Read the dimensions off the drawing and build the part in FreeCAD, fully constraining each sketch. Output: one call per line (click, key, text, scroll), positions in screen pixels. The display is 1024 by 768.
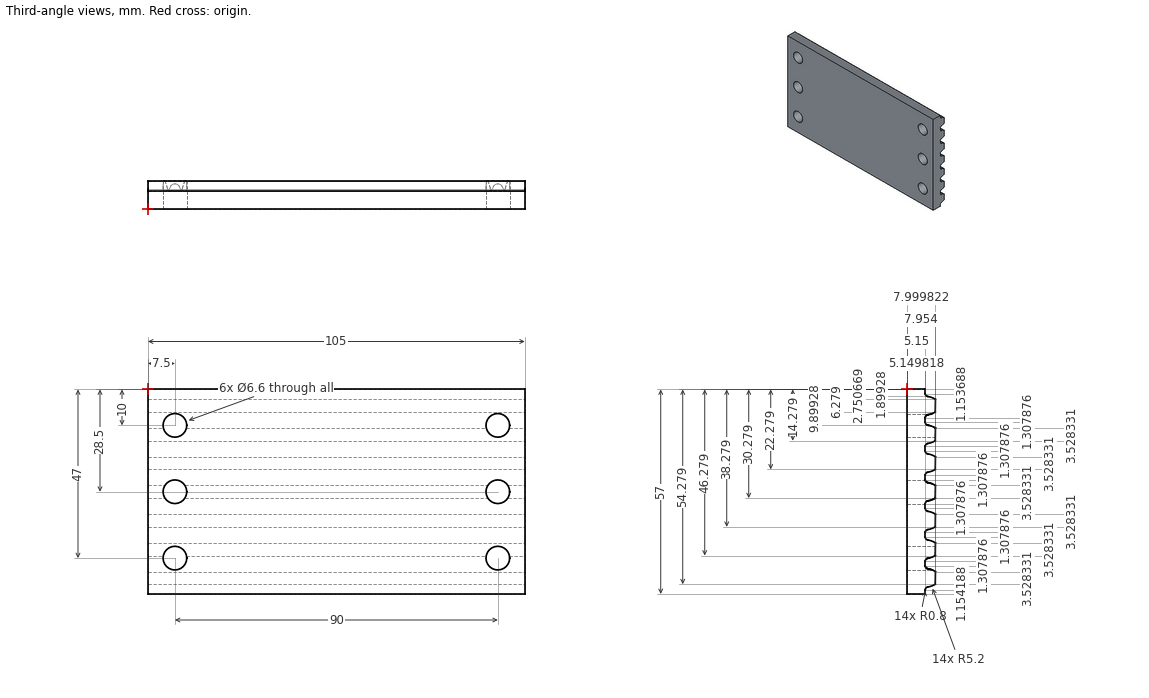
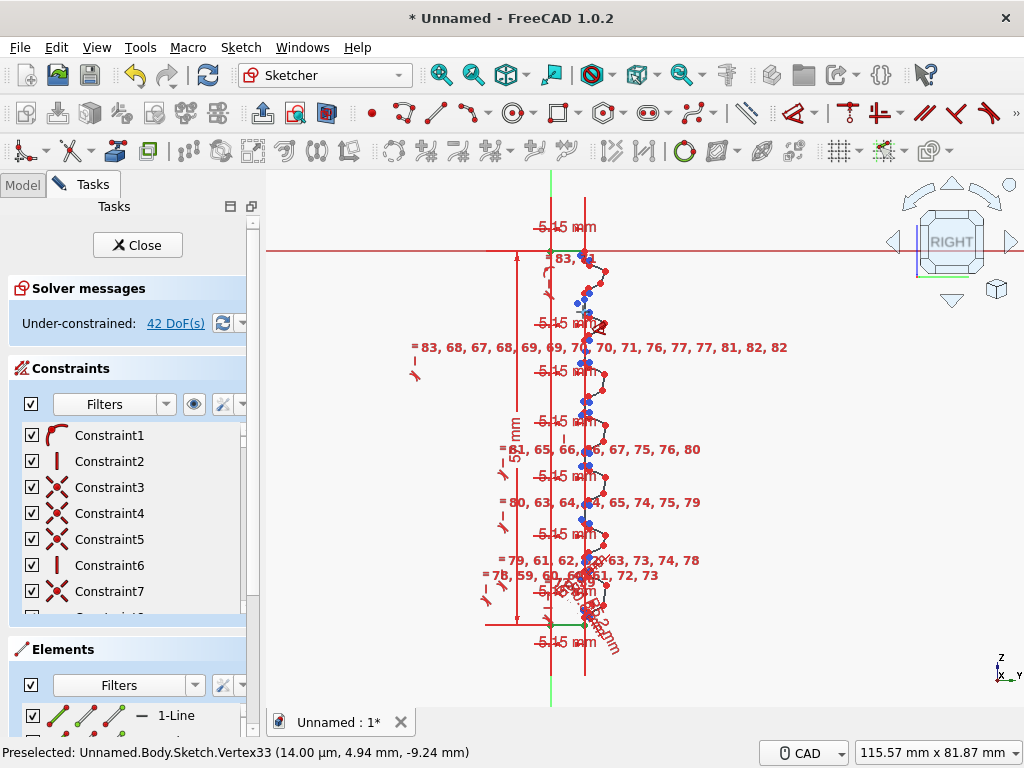
click(603, 605)
click(577, 217)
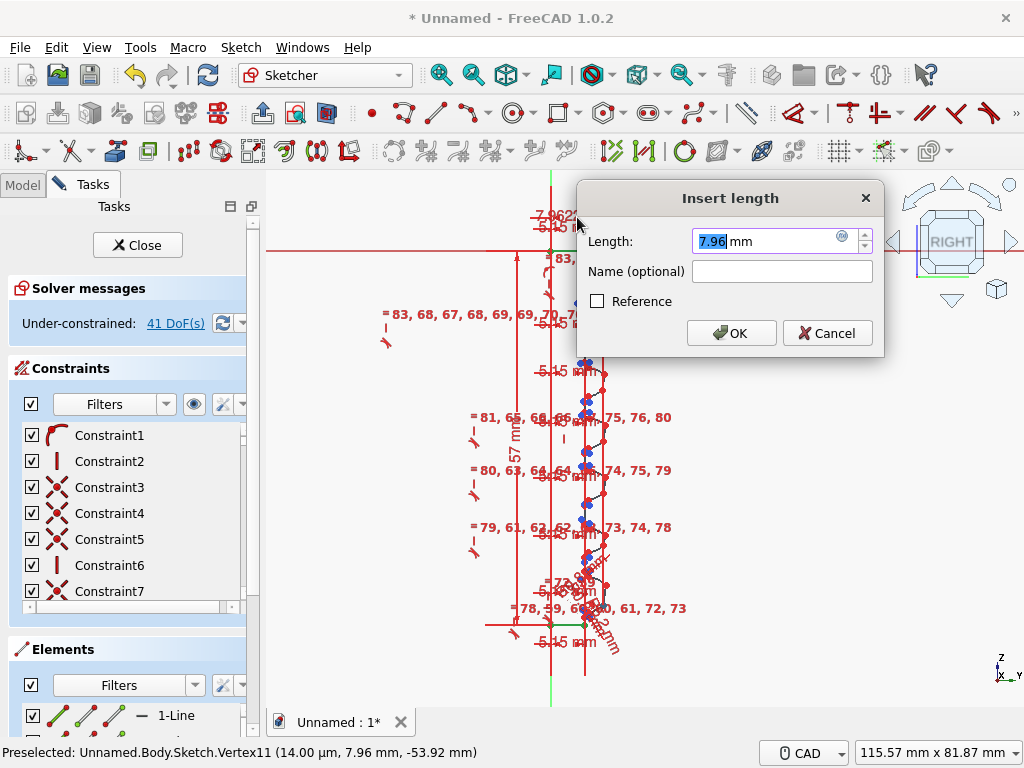
text(7.954)
key(Return)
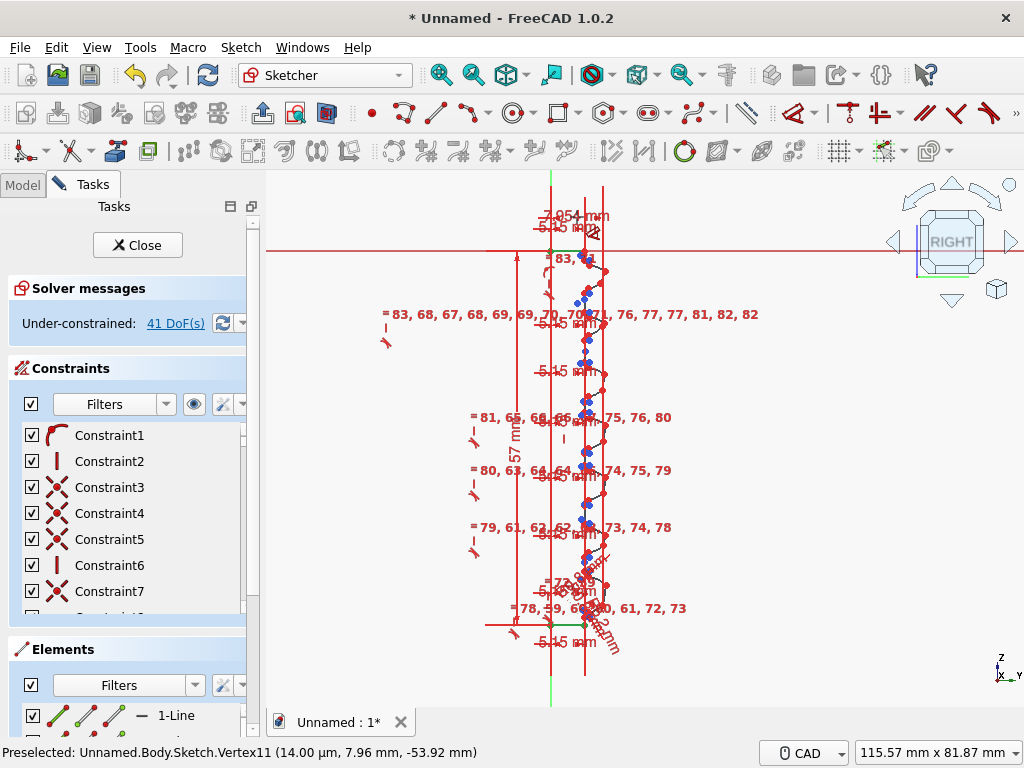
click(603, 546)
click(577, 676)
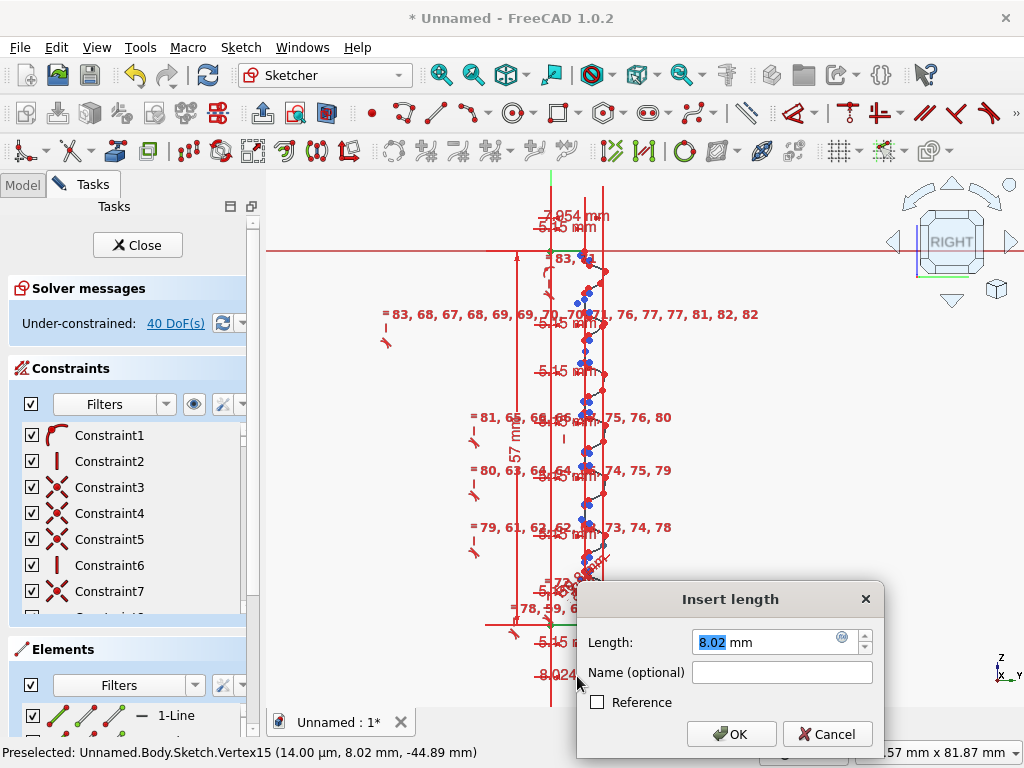
text(7.954)
key(Return)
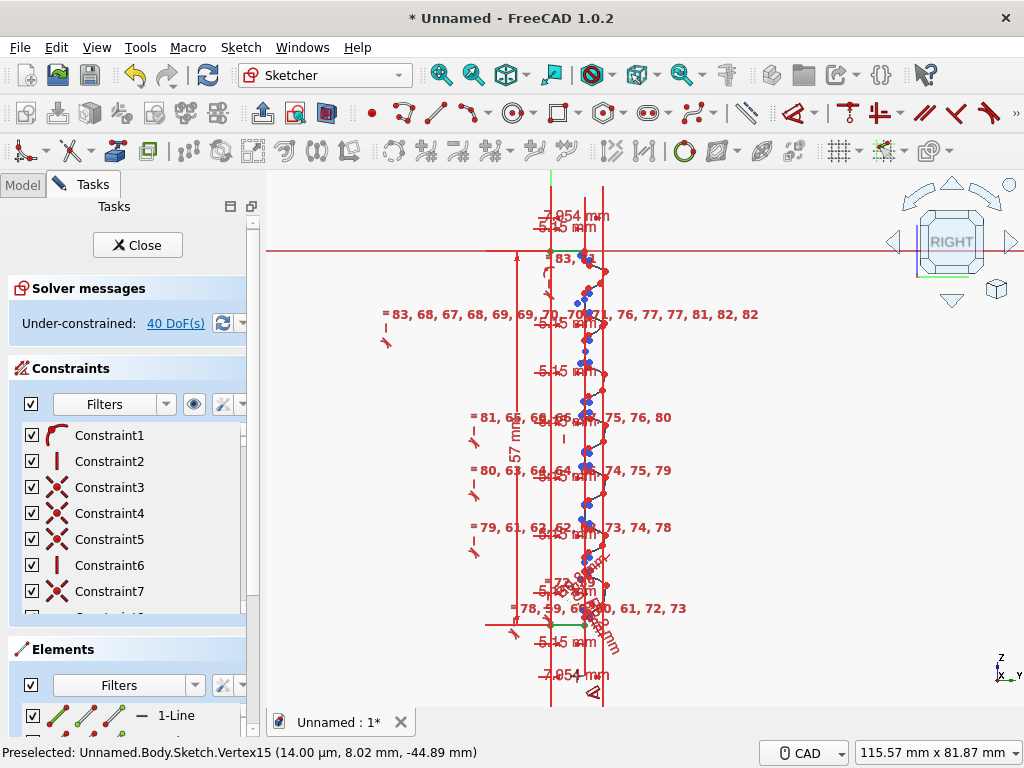
click(603, 493)
click(577, 551)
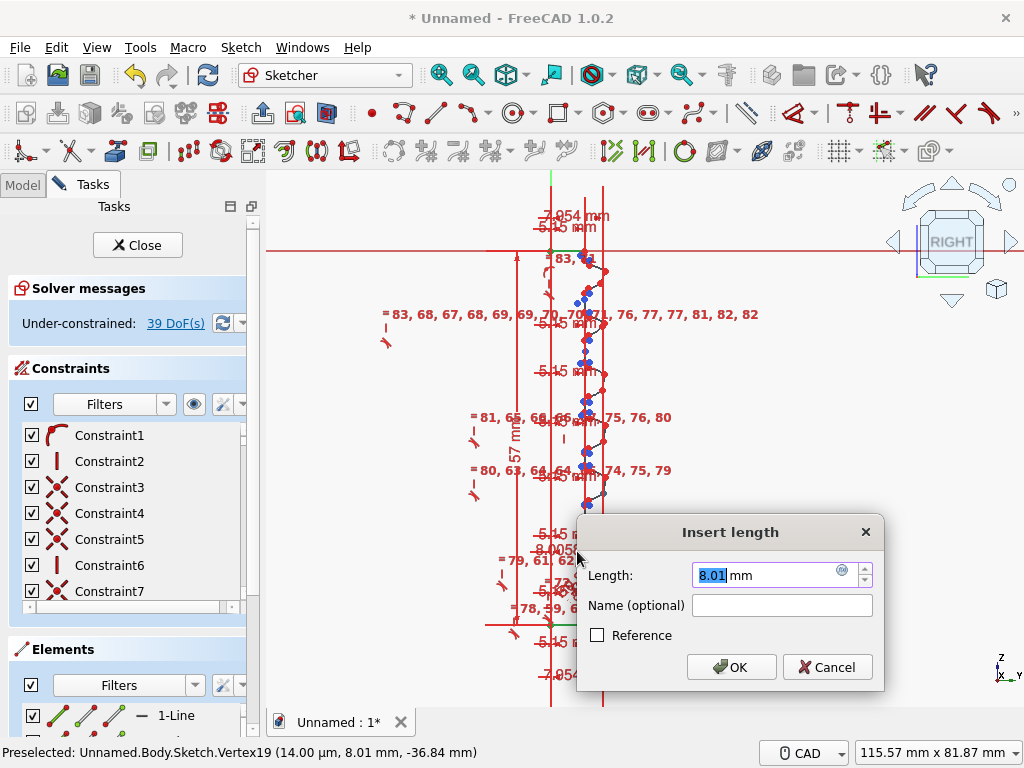
text(7.954)
key(Return)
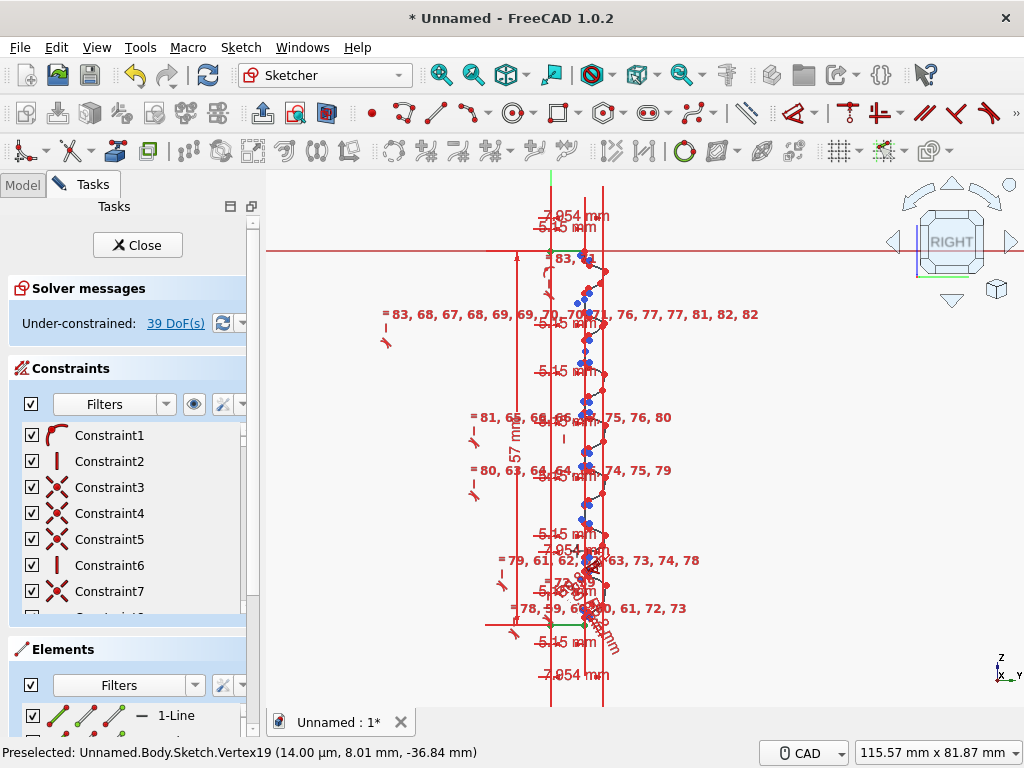
click(603, 442)
click(577, 500)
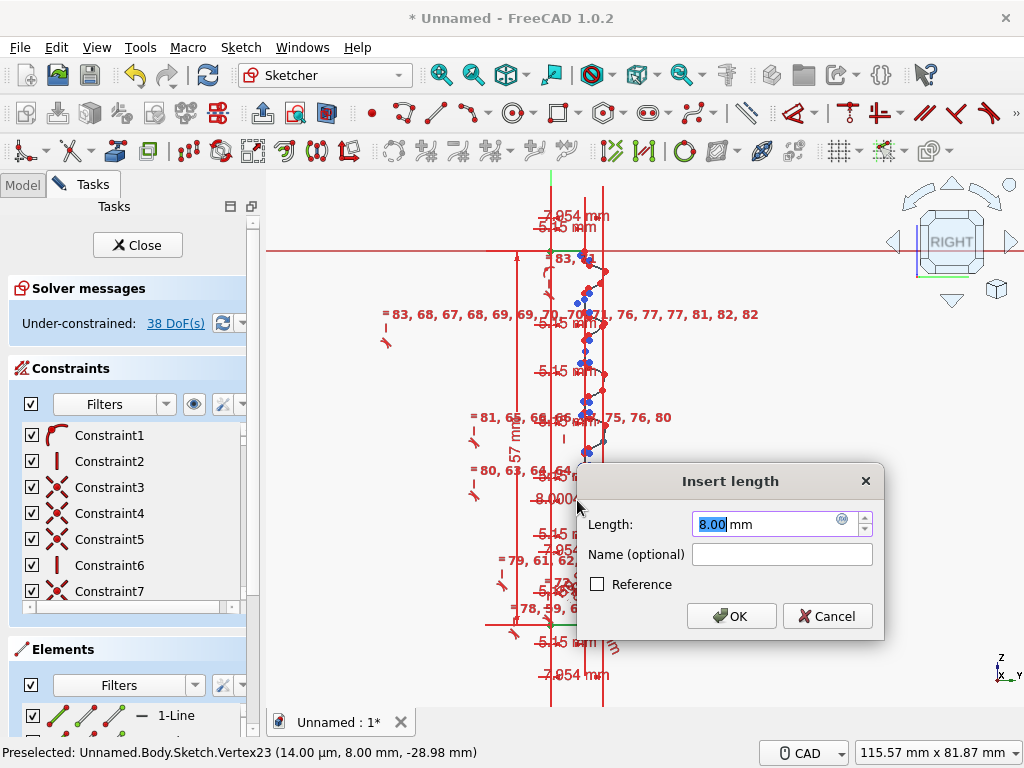
text(7.954)
key(Return)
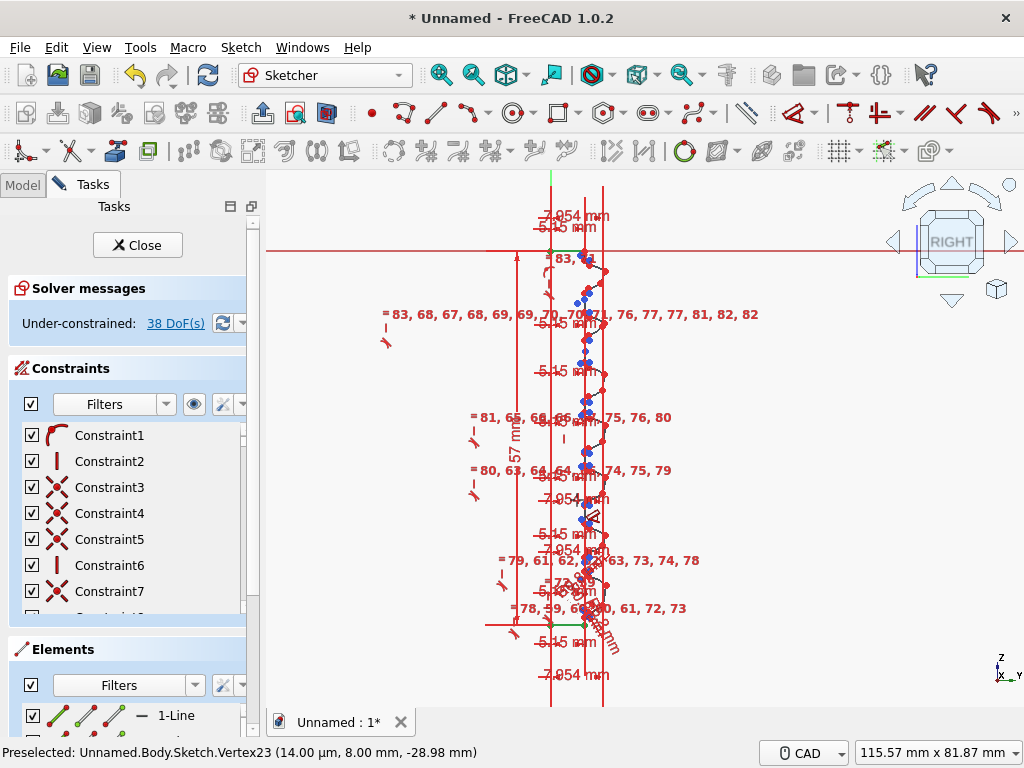
click(602, 390)
click(576, 448)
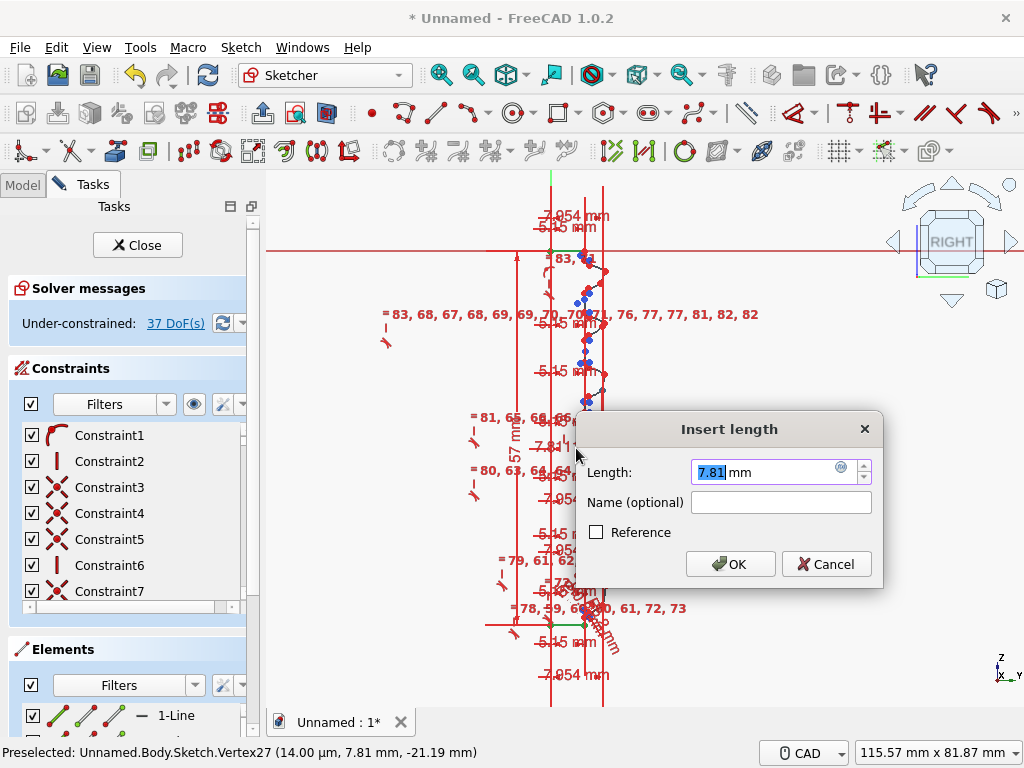
text(7.954)
key(Return)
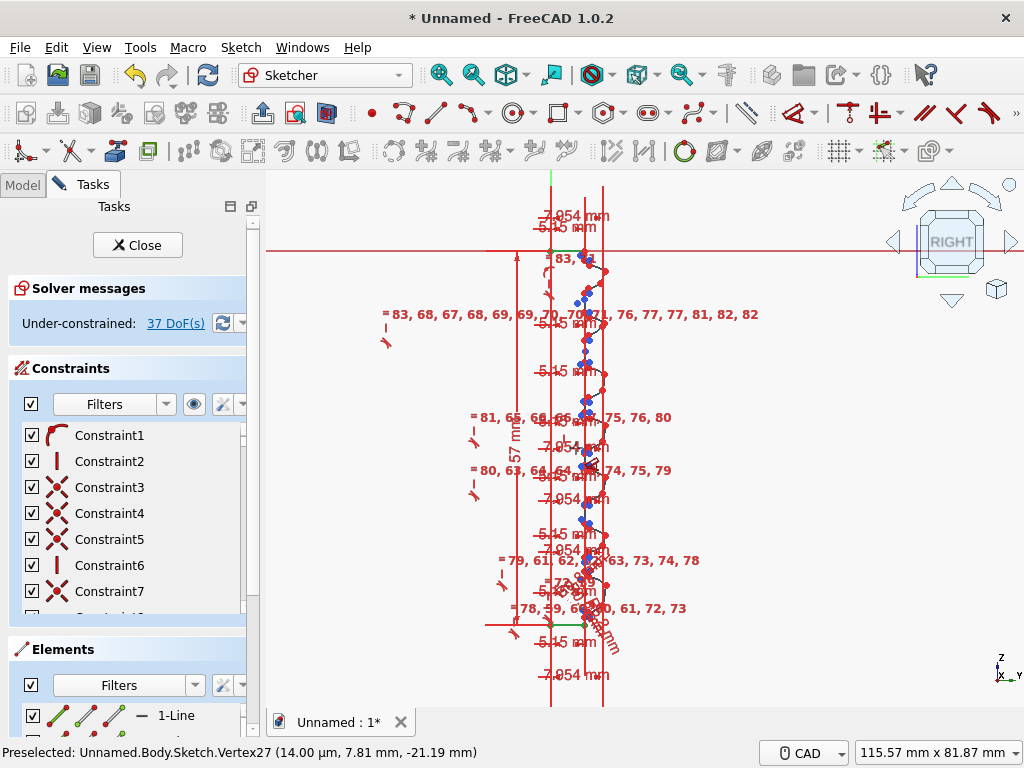
scroll(603, 326, up, 7)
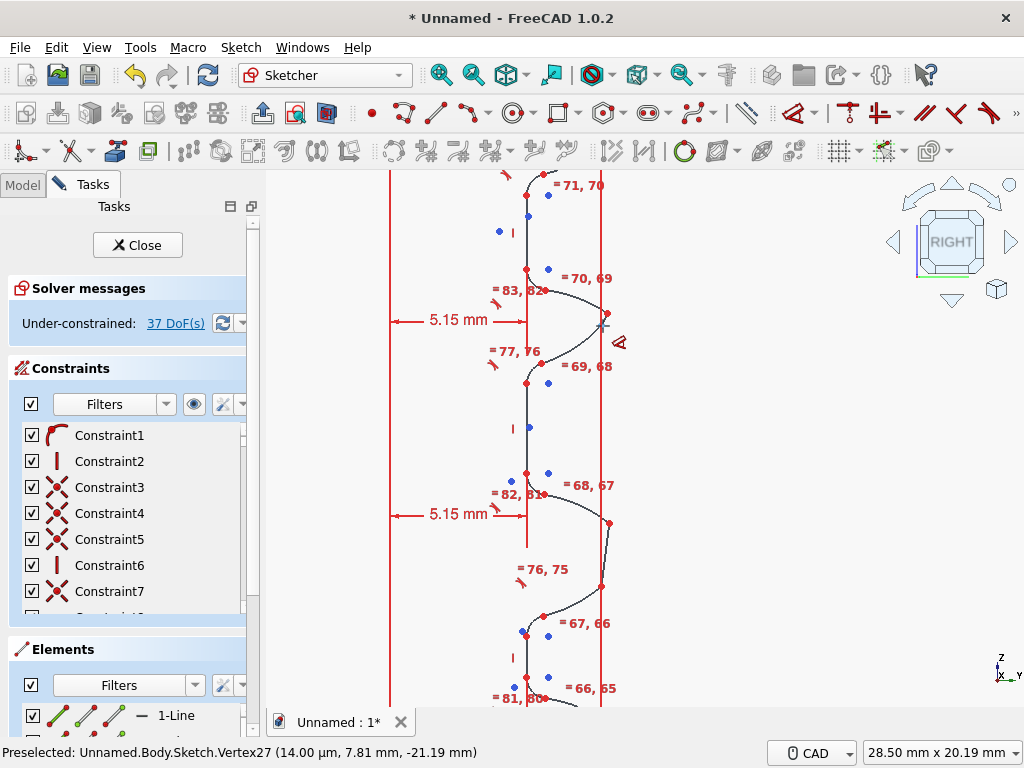
click(601, 325)
click(496, 359)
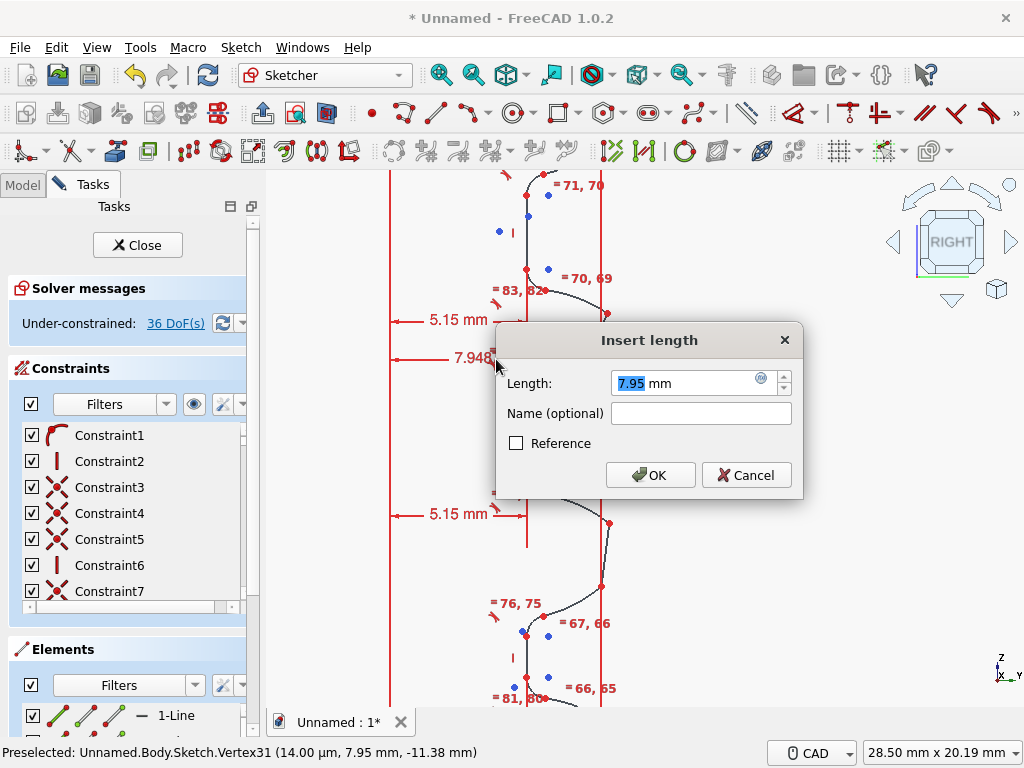
text(7.954)
key(Return)